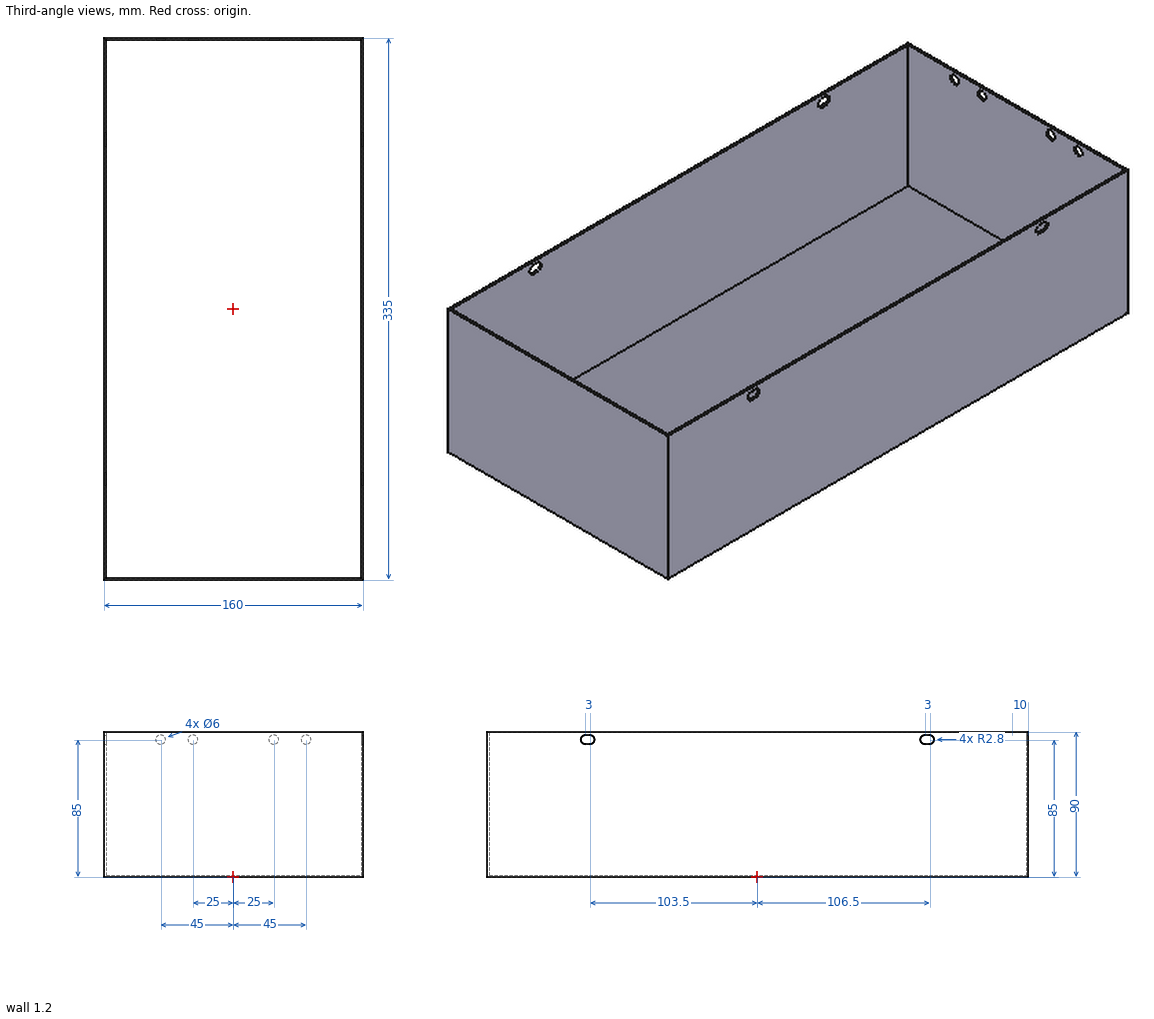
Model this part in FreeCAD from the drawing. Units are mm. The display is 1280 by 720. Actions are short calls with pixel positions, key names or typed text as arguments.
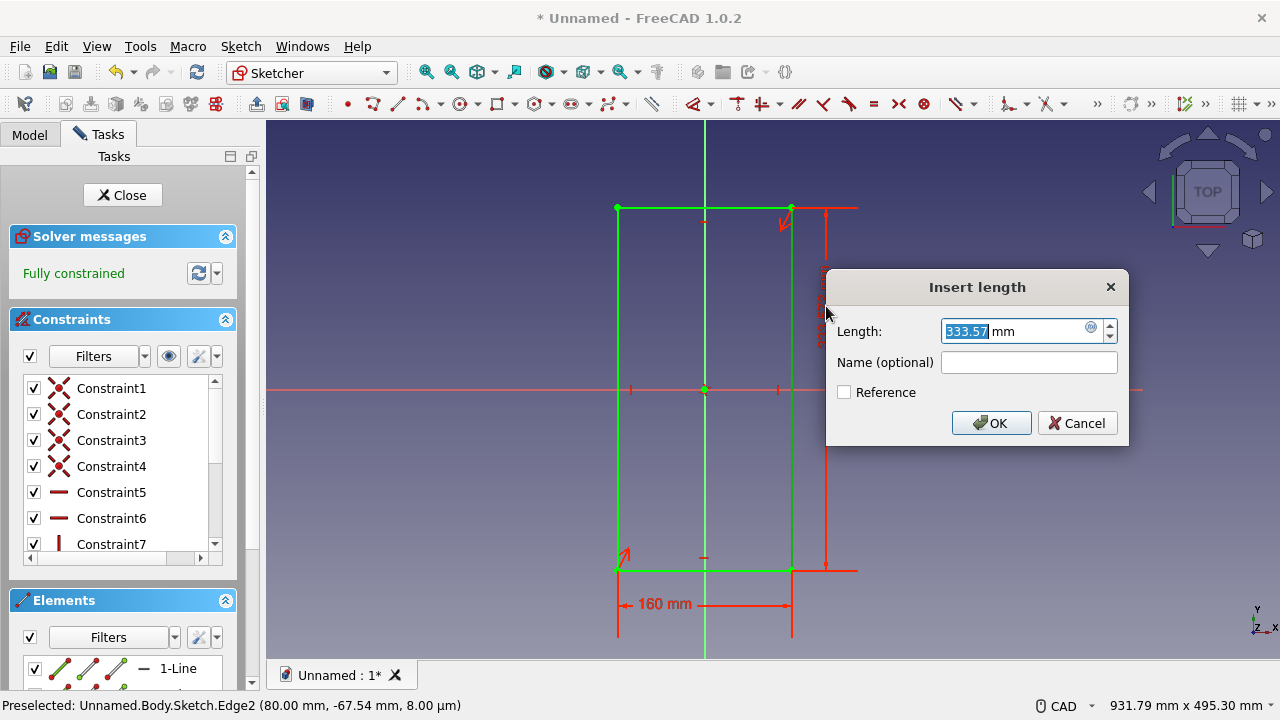
text(335)
key(Return)
key(Escape)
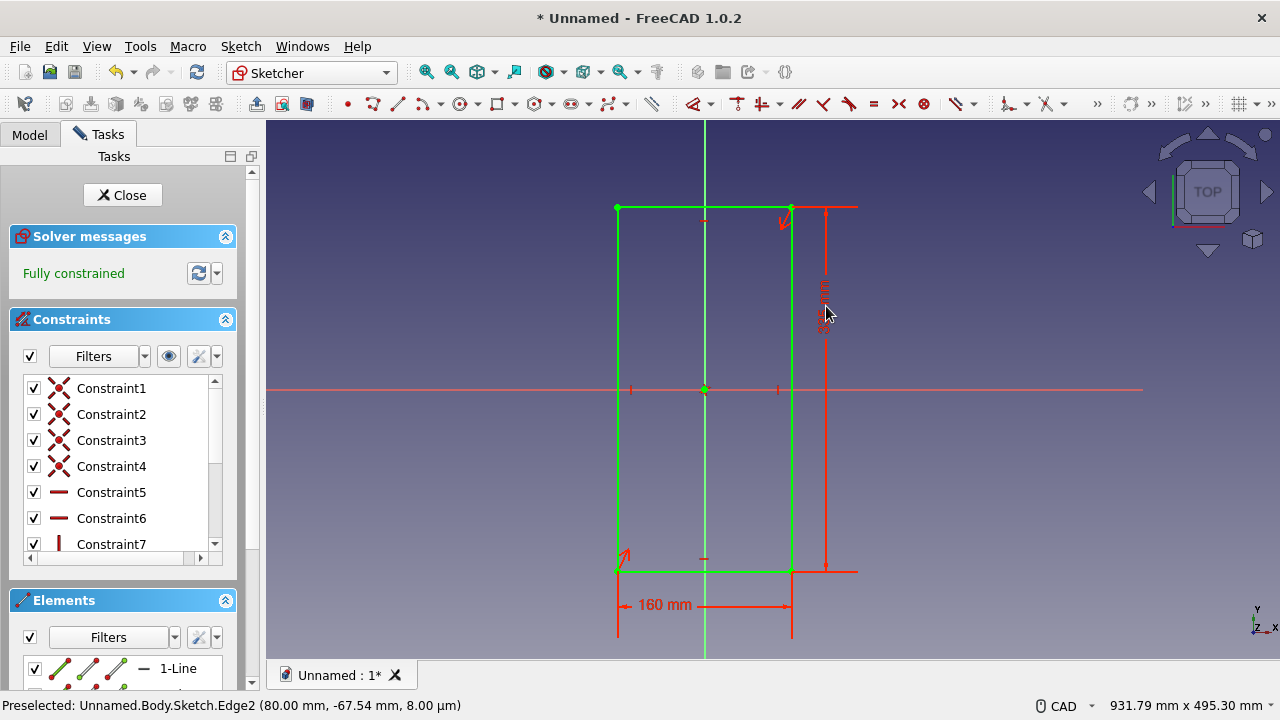
click(123, 195)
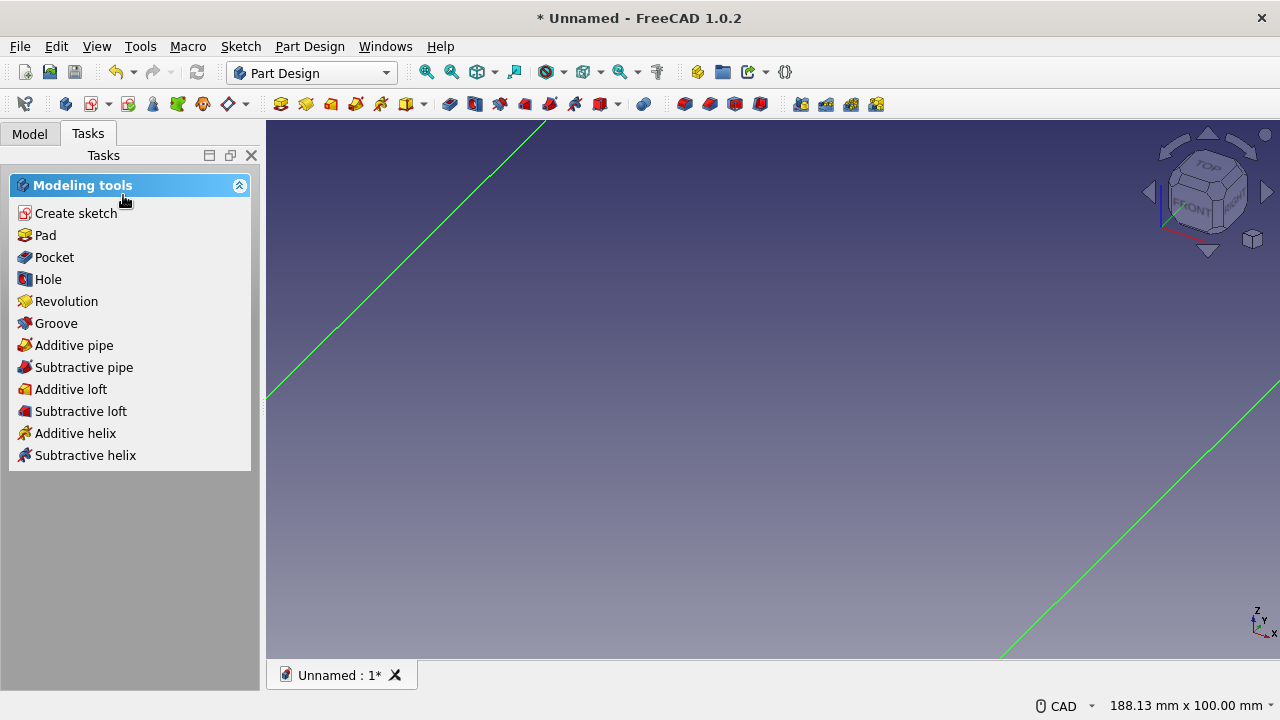
click(281, 104)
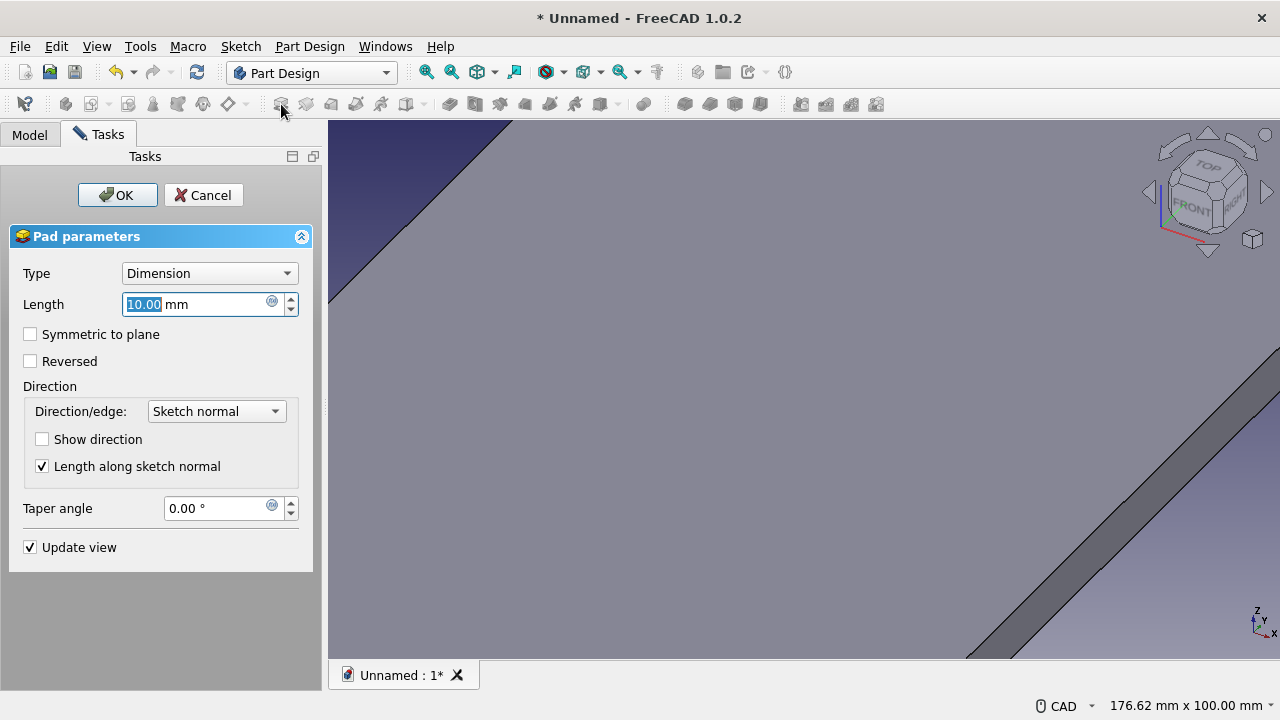
text(90)
key(Tab)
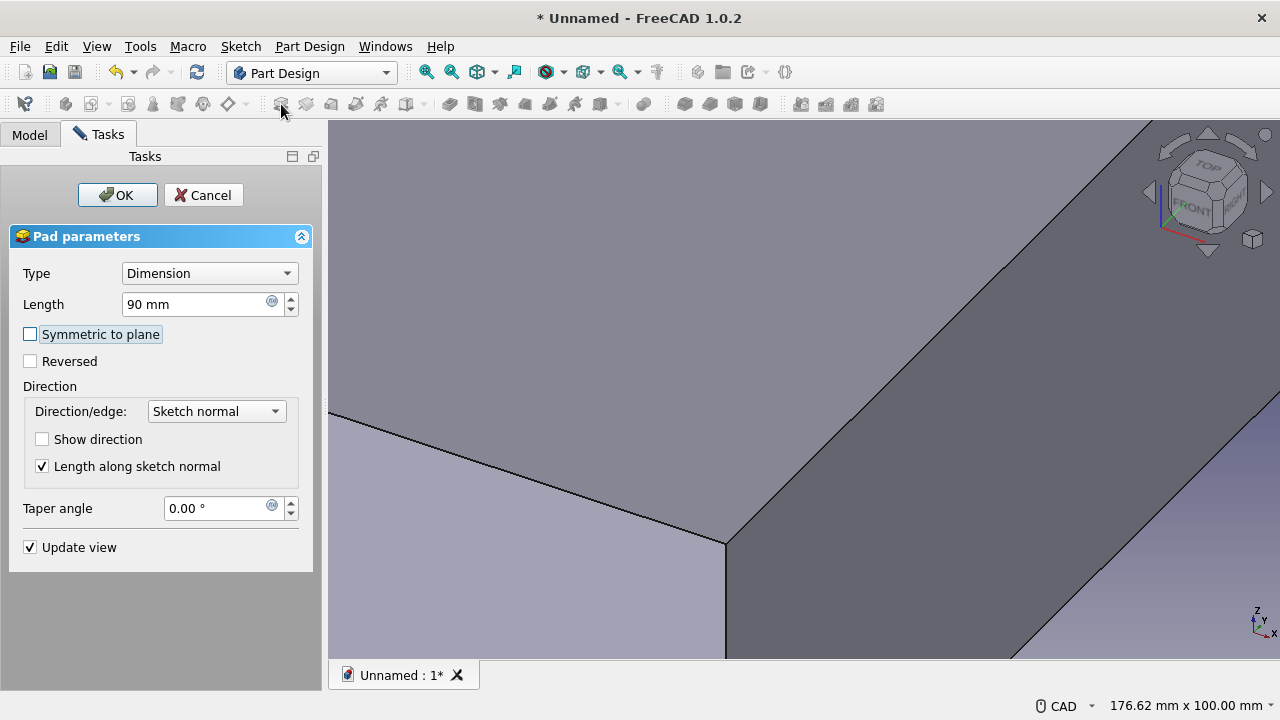
click(118, 195)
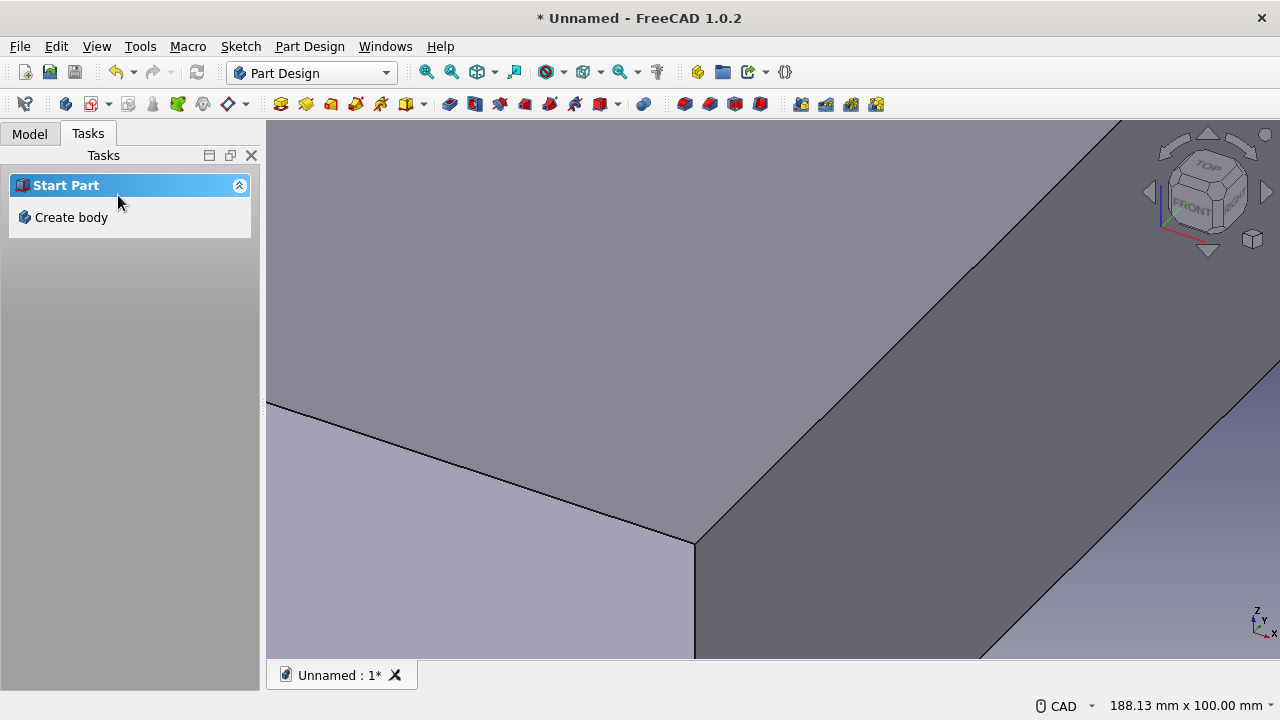
click(427, 72)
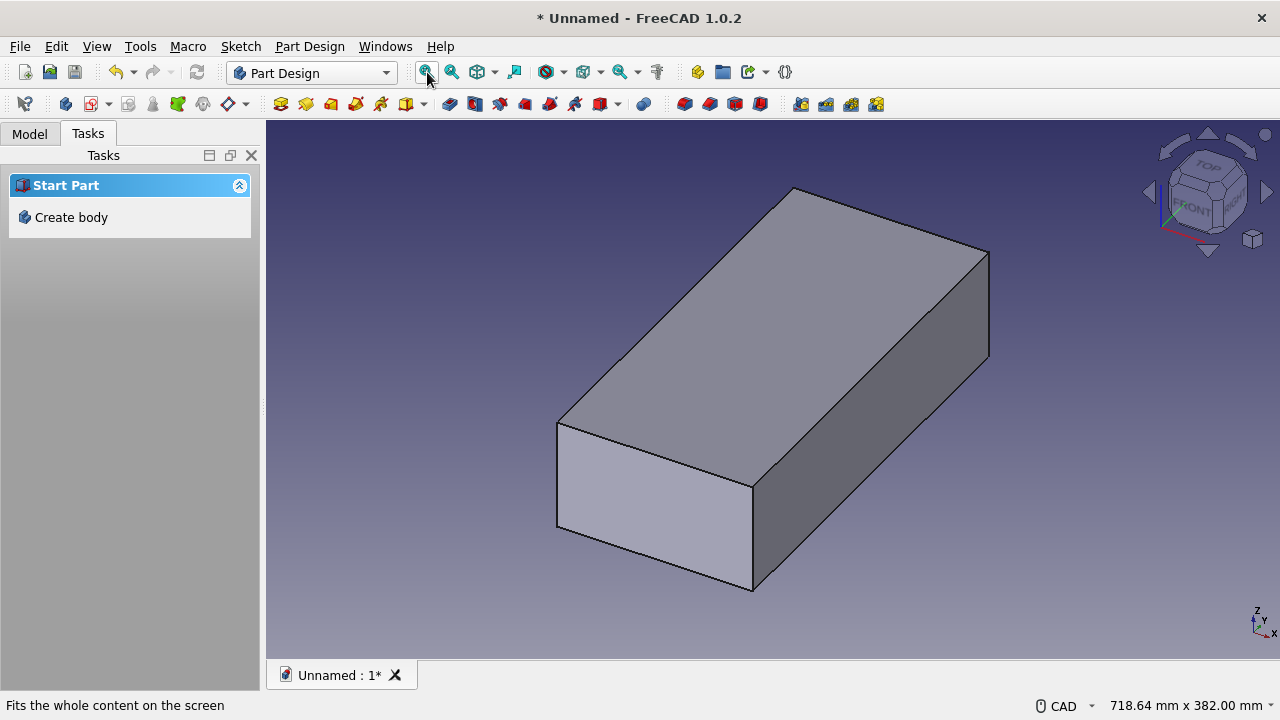
click(807, 303)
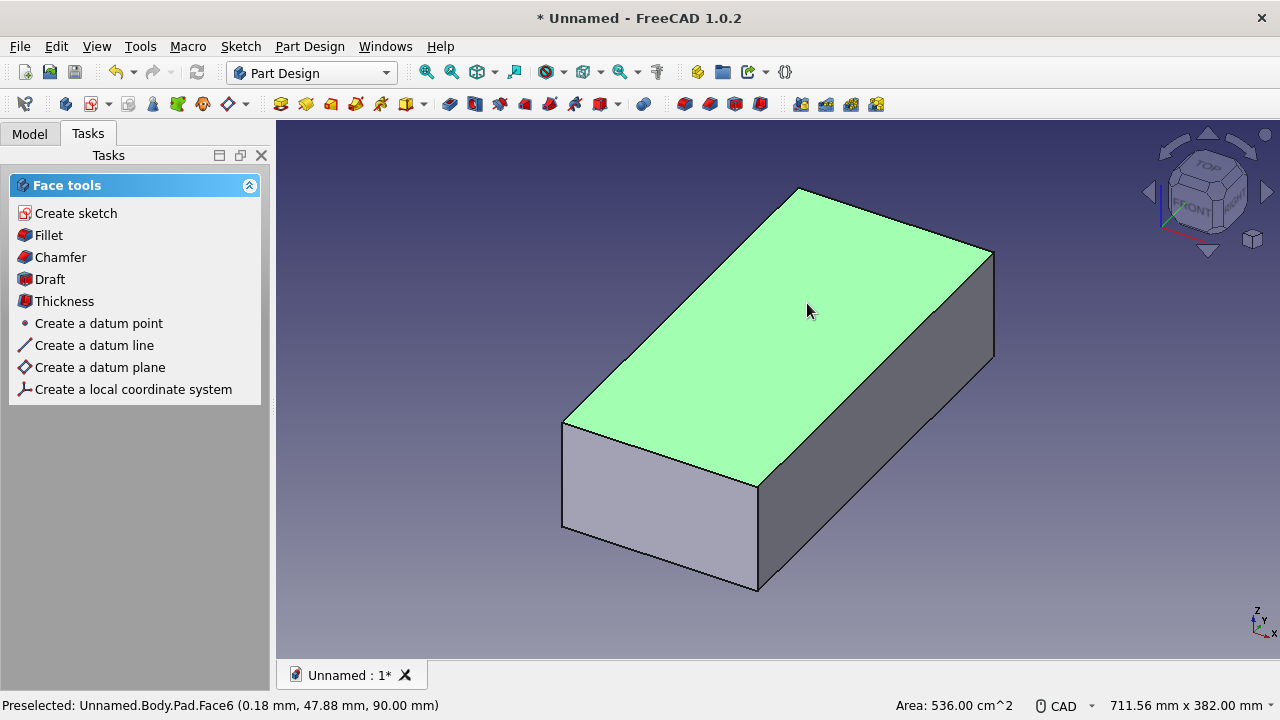
click(760, 104)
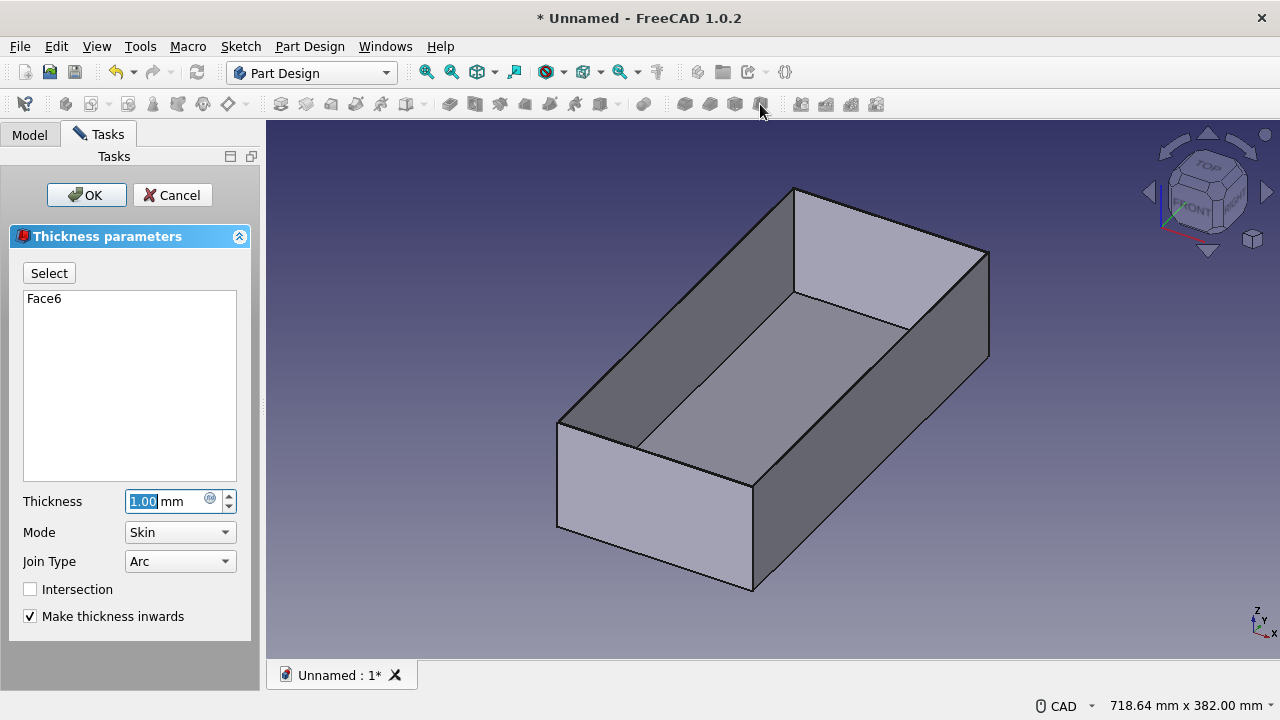
text(1.2)
key(Tab)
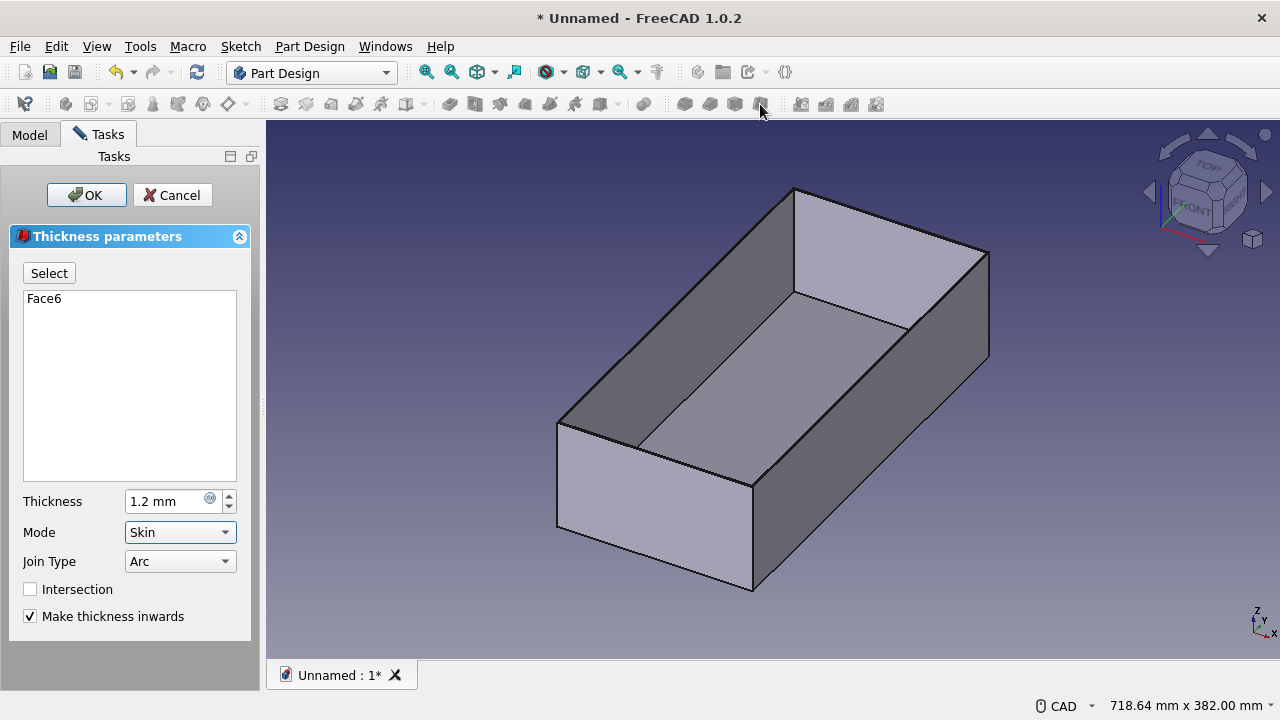
click(181, 562)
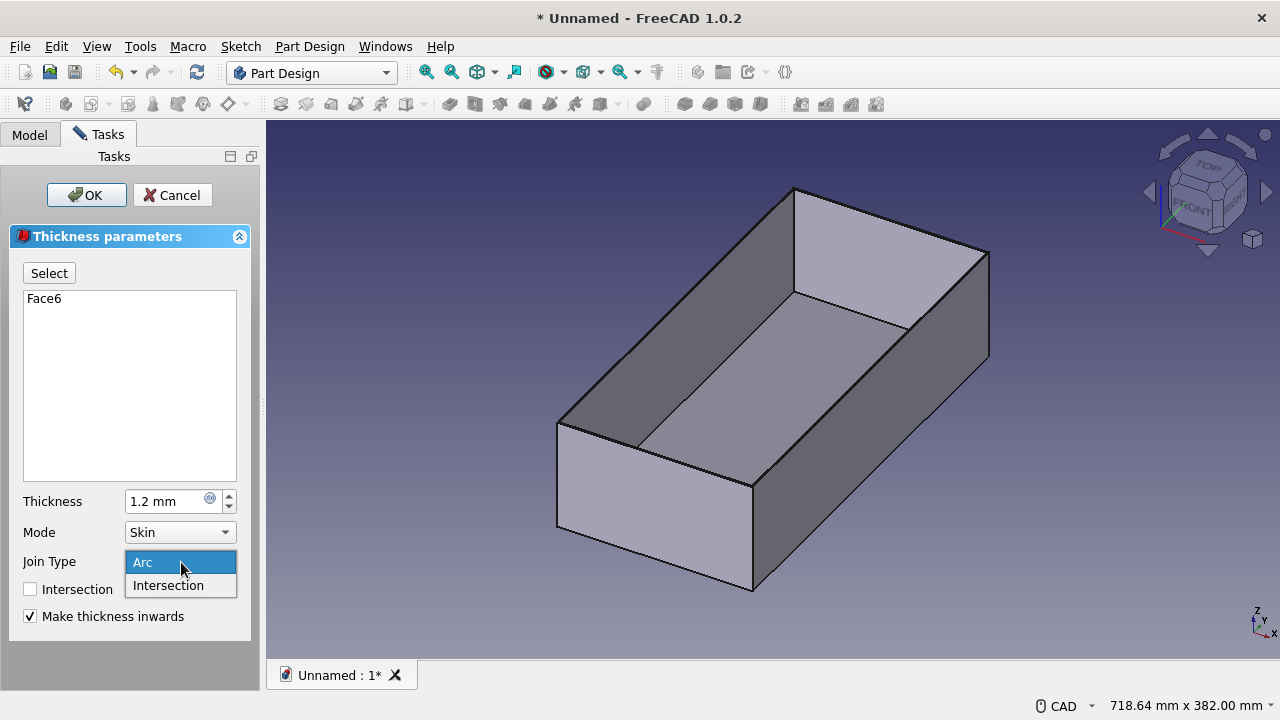
click(179, 586)